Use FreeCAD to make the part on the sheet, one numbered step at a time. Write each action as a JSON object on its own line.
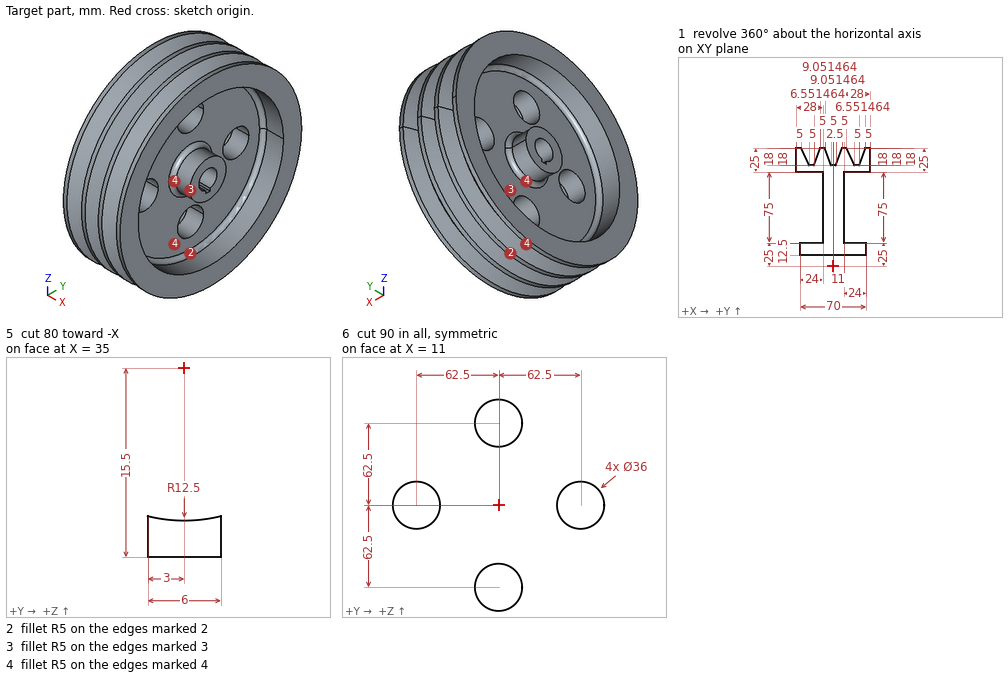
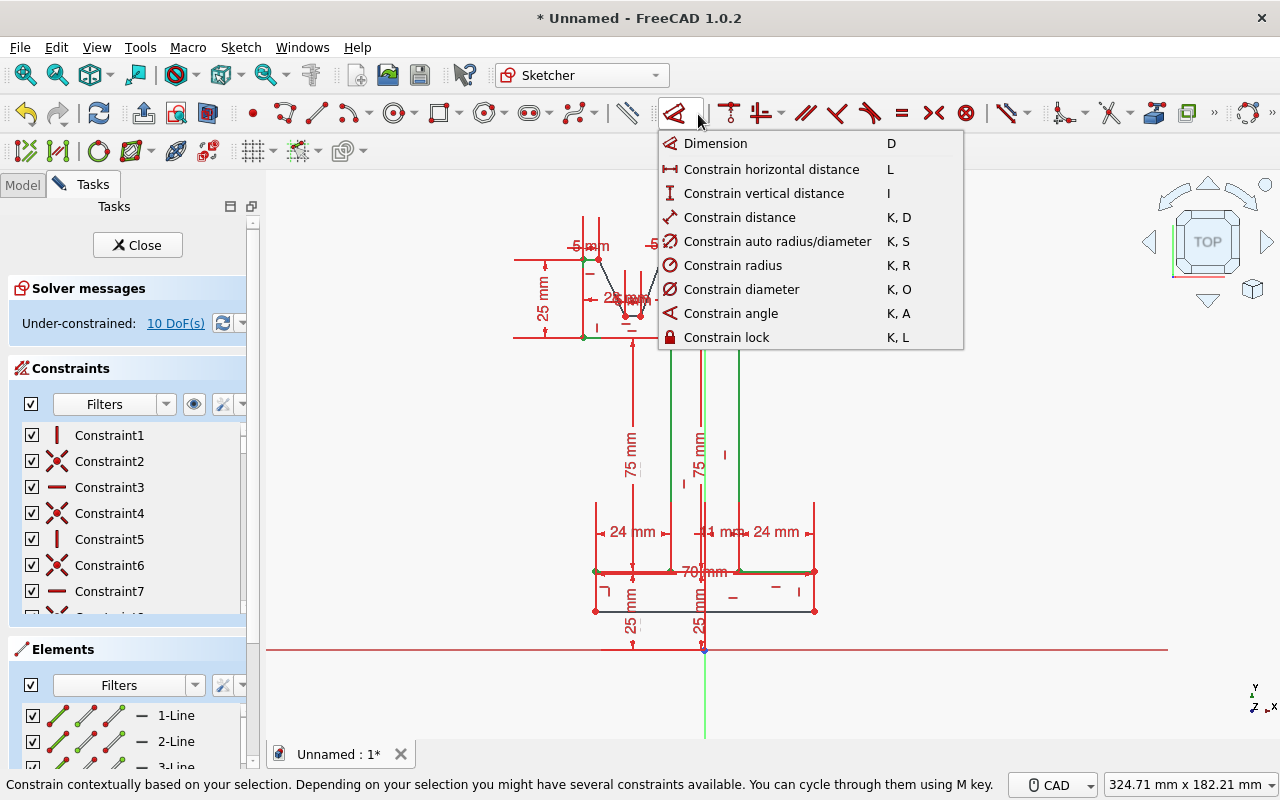
{"action": "left_click", "coordinate": [811, 193]}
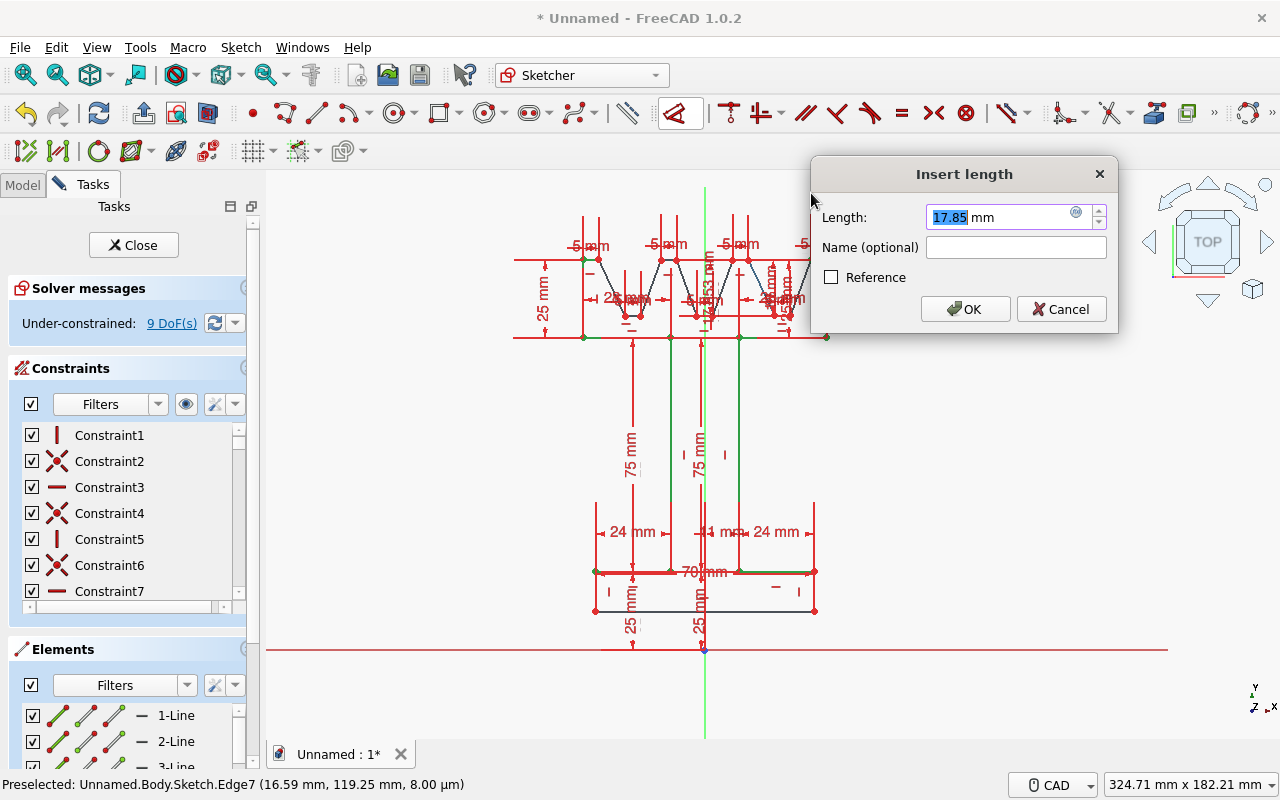
{"action": "type", "text": "18"}
{"action": "key", "text": "Return"}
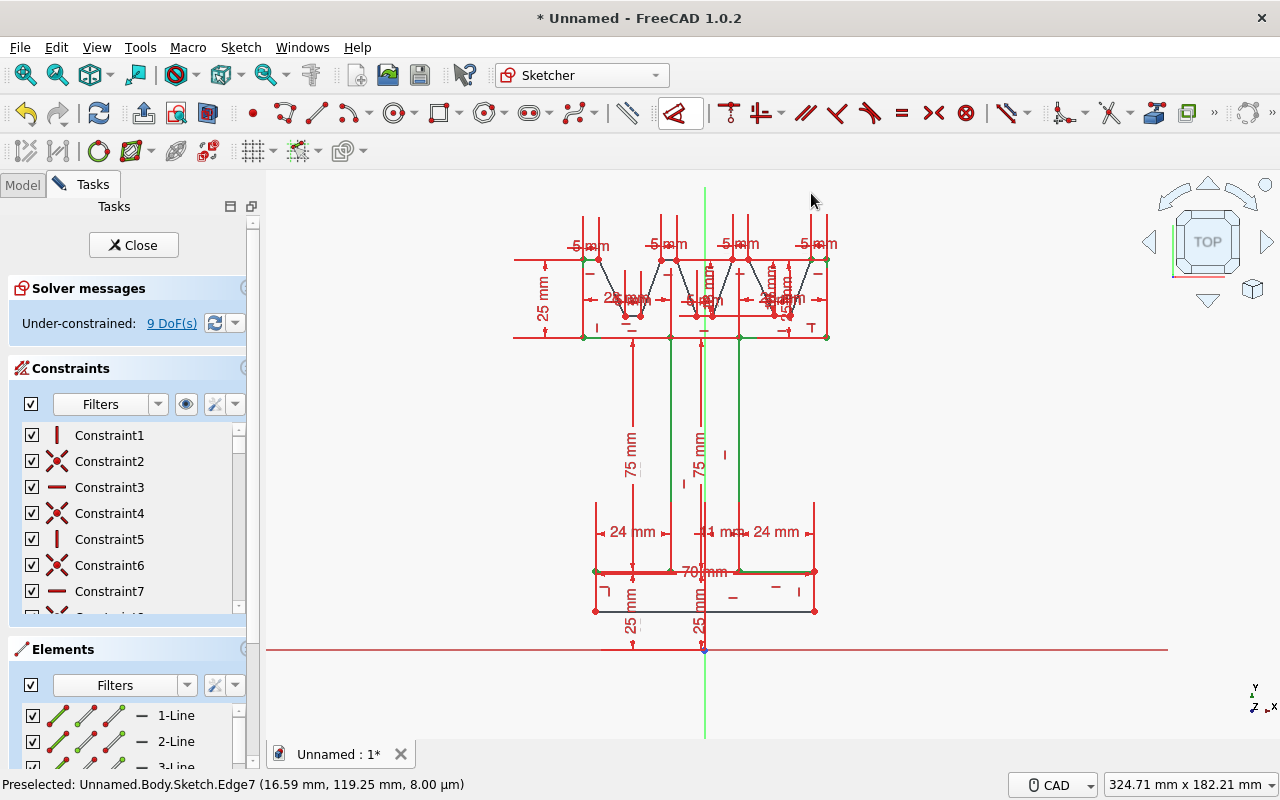
{"action": "left_click", "coordinate": [727, 277]}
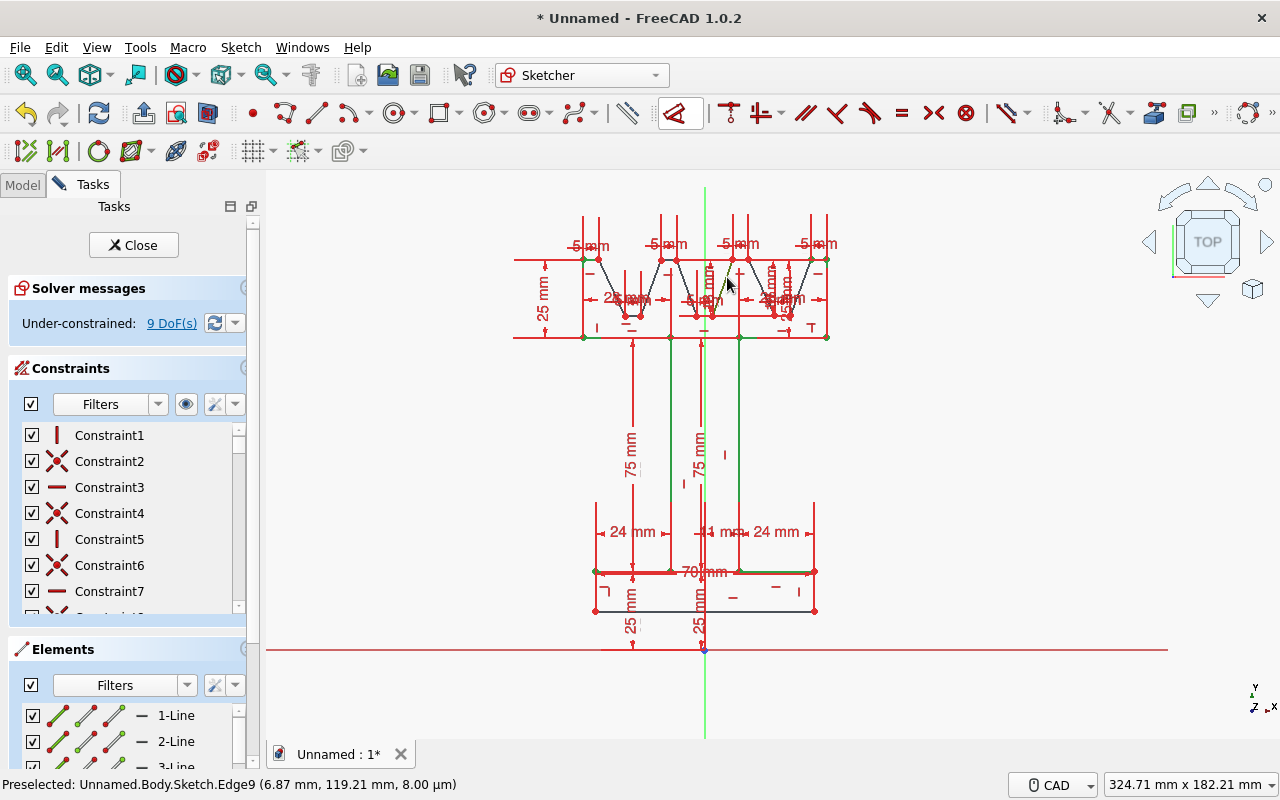
{"action": "key", "text": "i"}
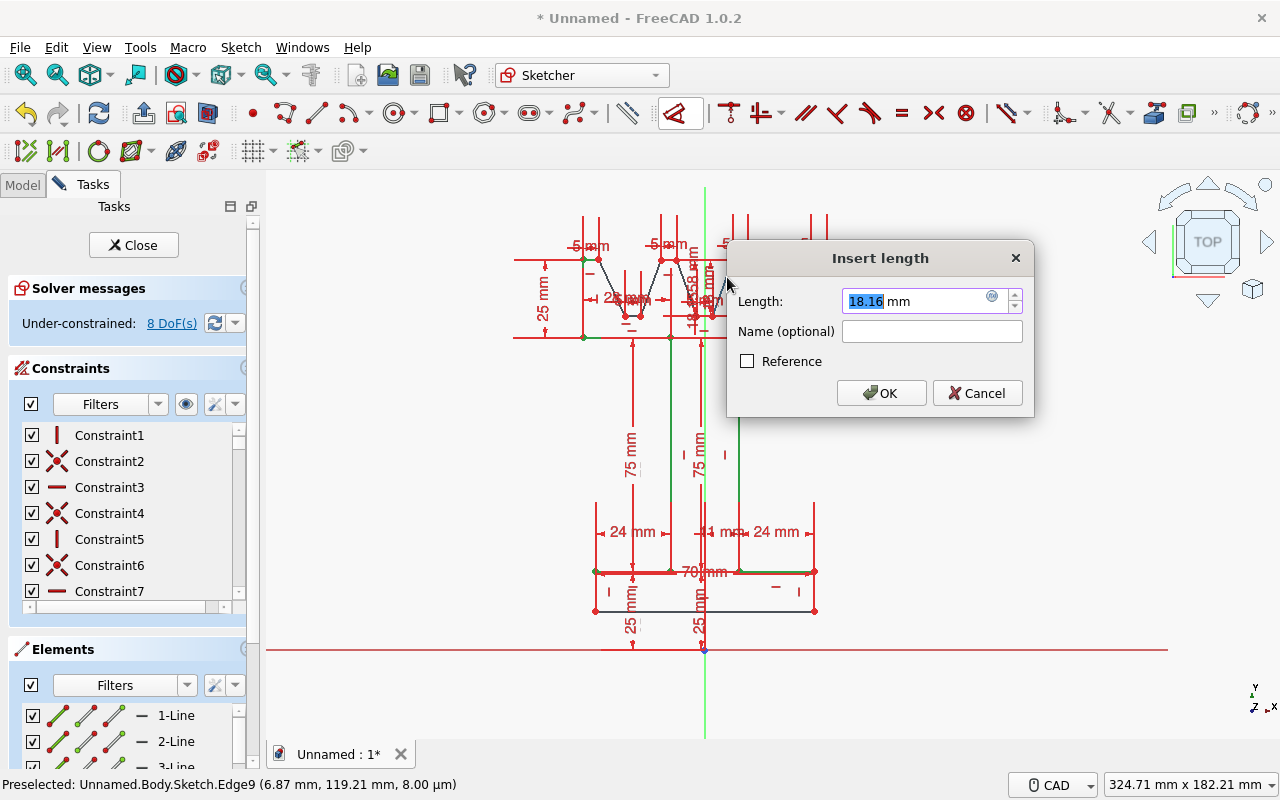
{"action": "type", "text": "18"}
{"action": "key", "text": "Return"}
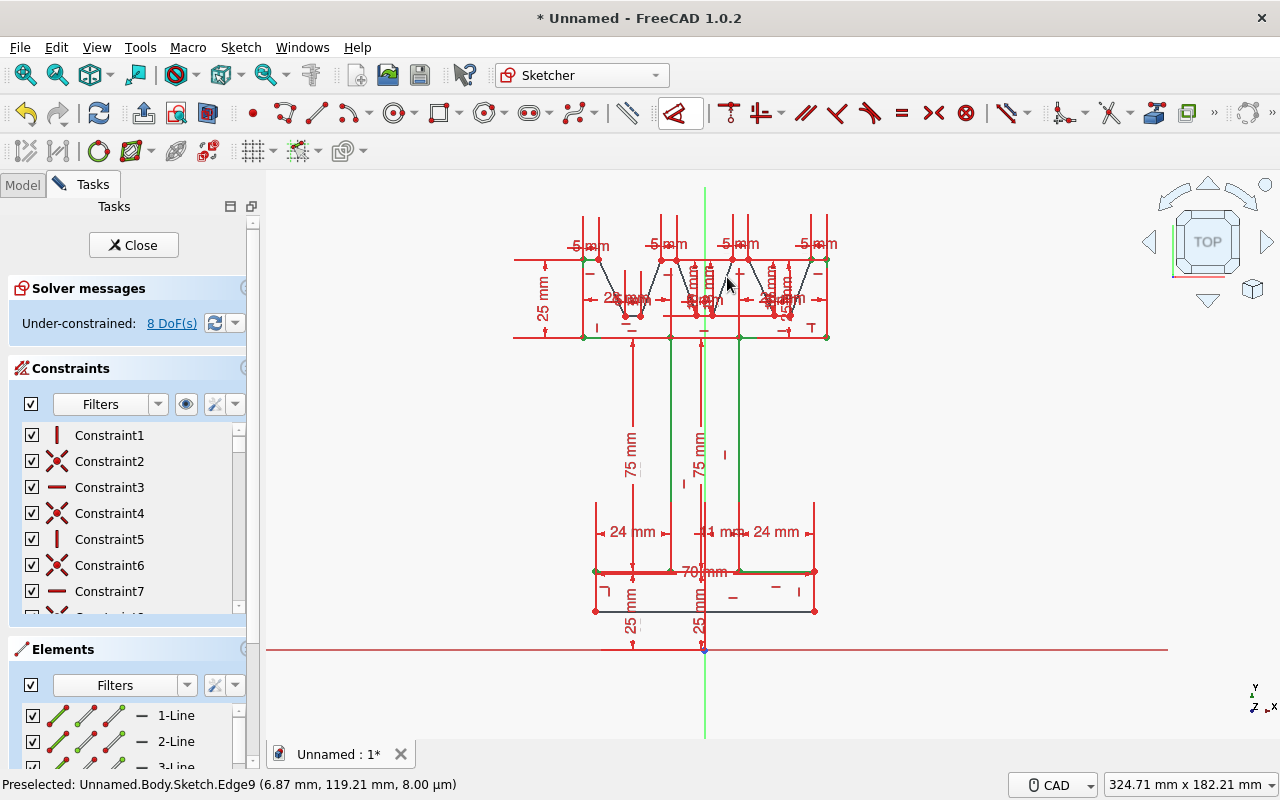
{"action": "left_click", "coordinate": [683, 277]}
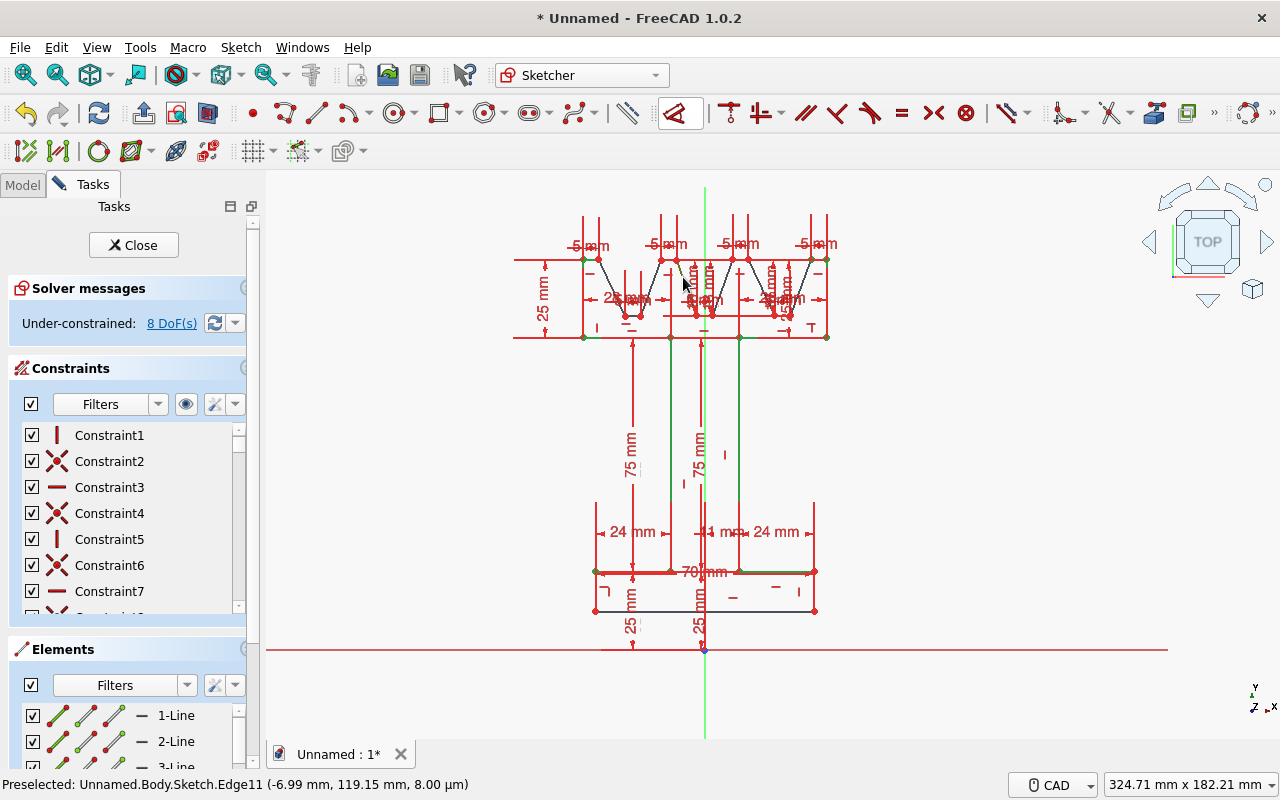
{"action": "key", "text": "i"}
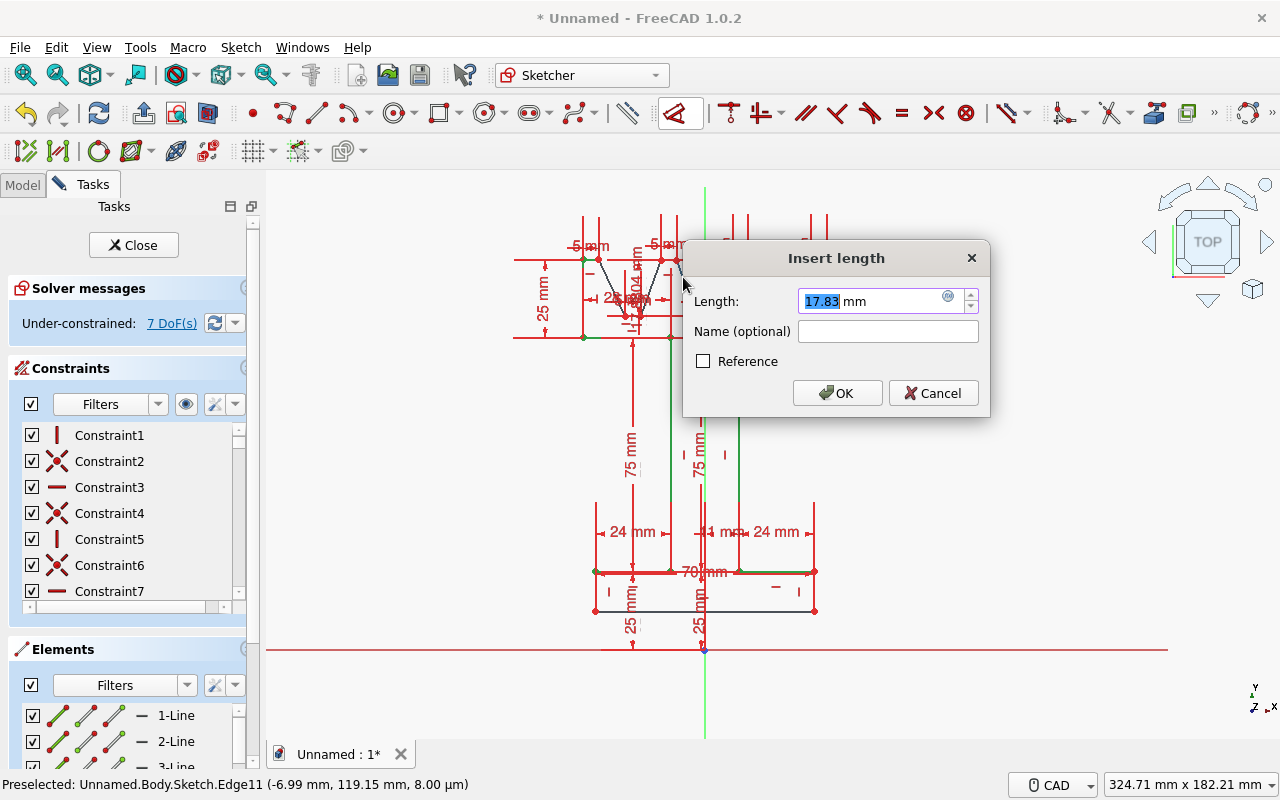
{"action": "type", "text": "18"}
{"action": "key", "text": "Return"}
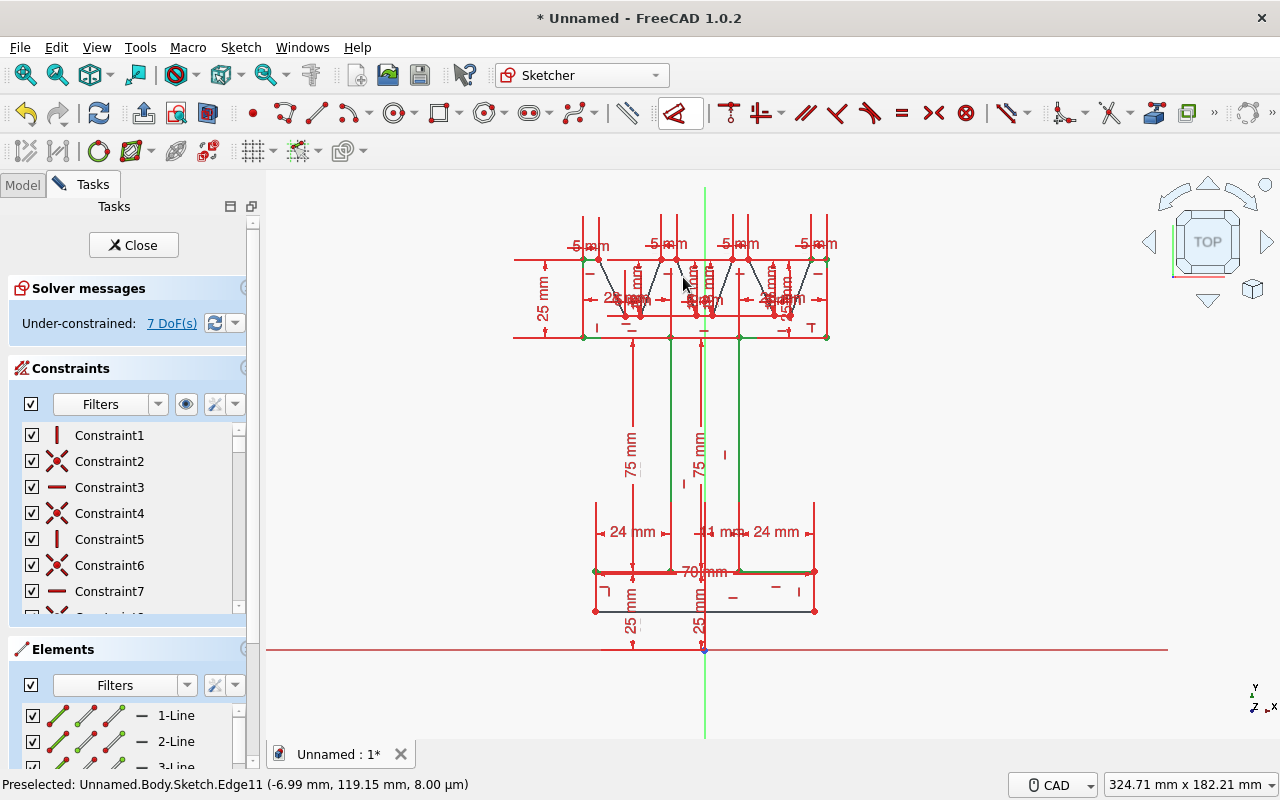
{"action": "left_click", "coordinate": [655, 277]}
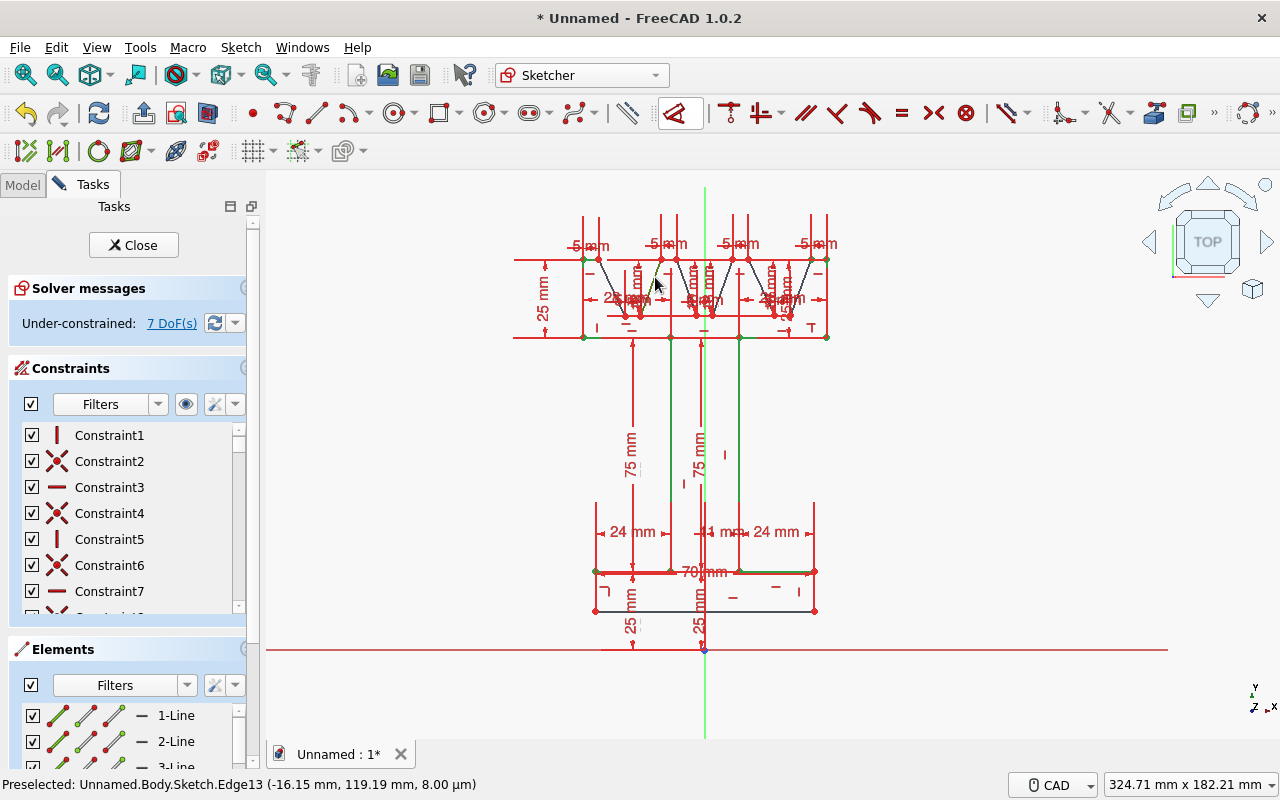
{"action": "left_click", "coordinate": [698, 114]}